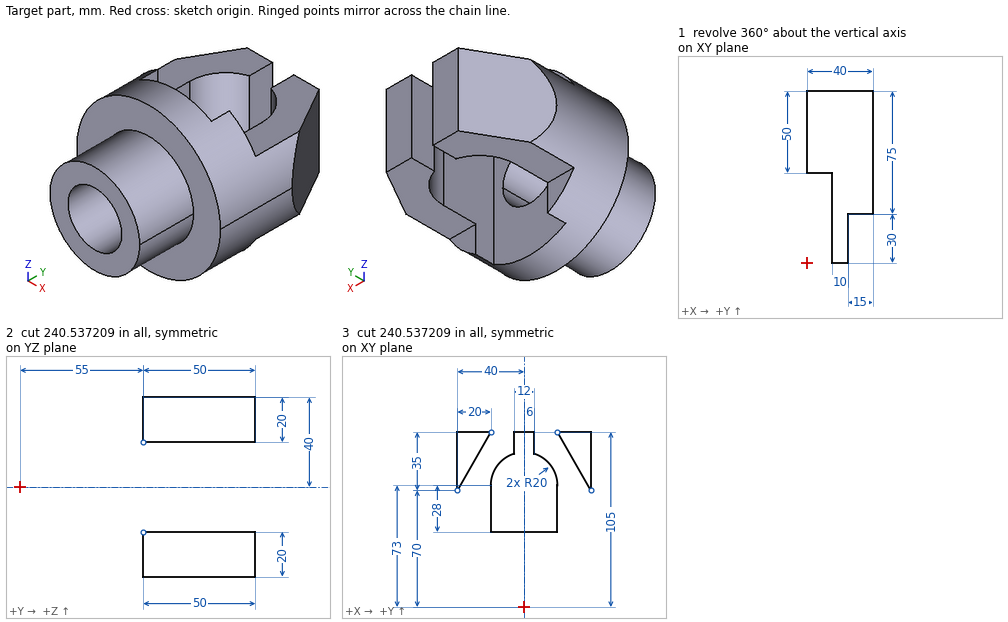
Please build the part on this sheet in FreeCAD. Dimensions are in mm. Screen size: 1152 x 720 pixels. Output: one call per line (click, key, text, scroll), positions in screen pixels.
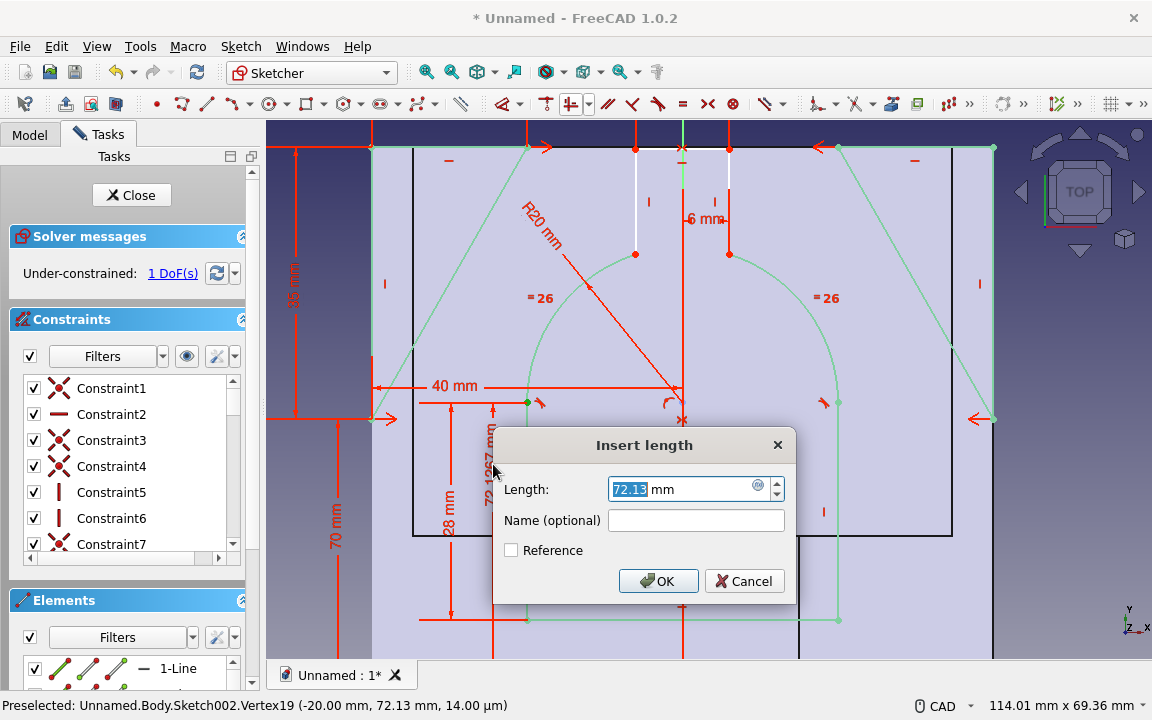
text(73)
key(Return)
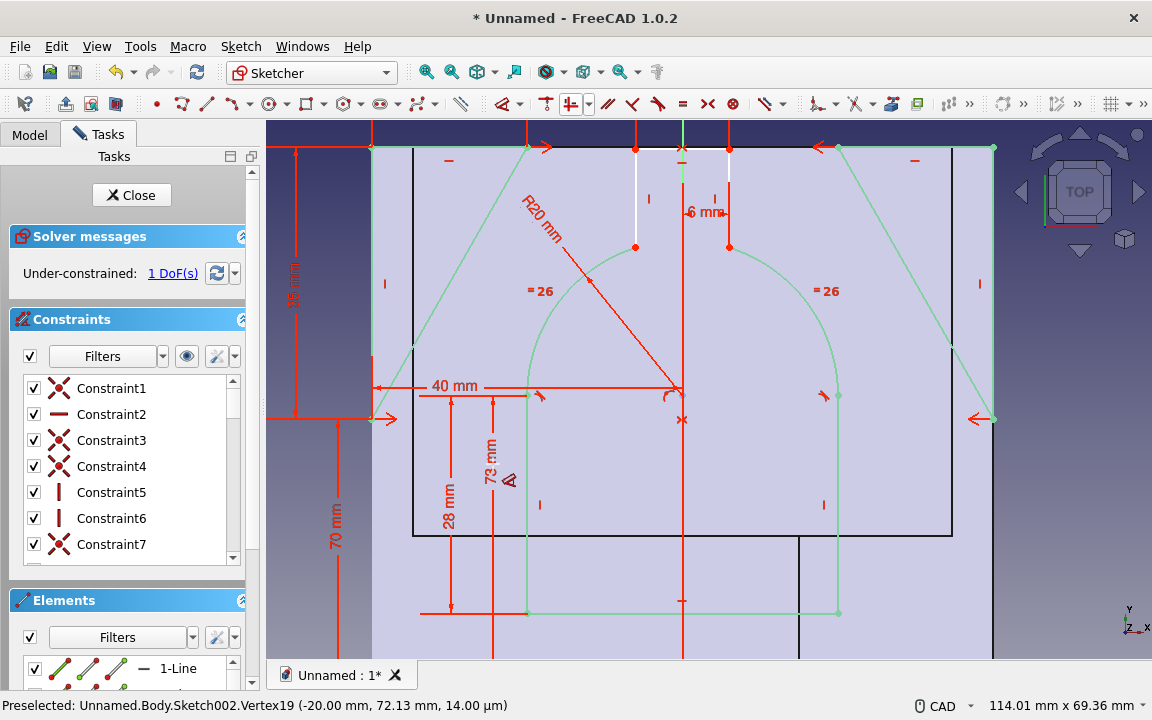
click(729, 149)
click(763, 390)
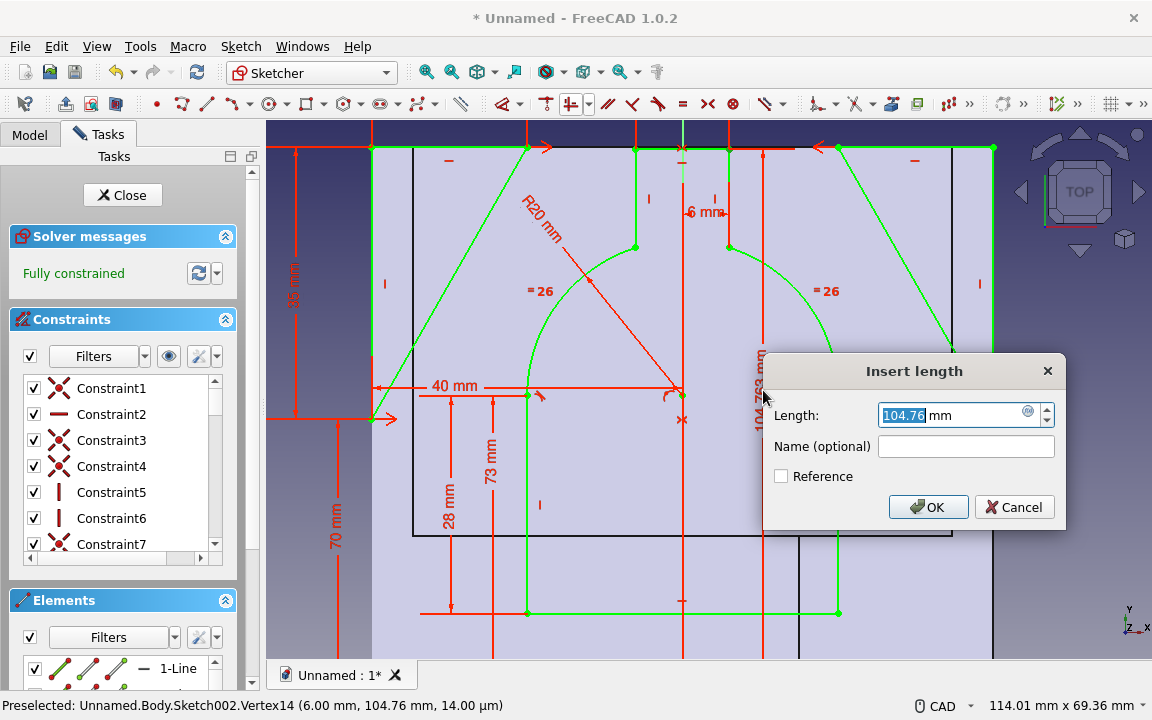
text(105)
key(Return)
key(Escape)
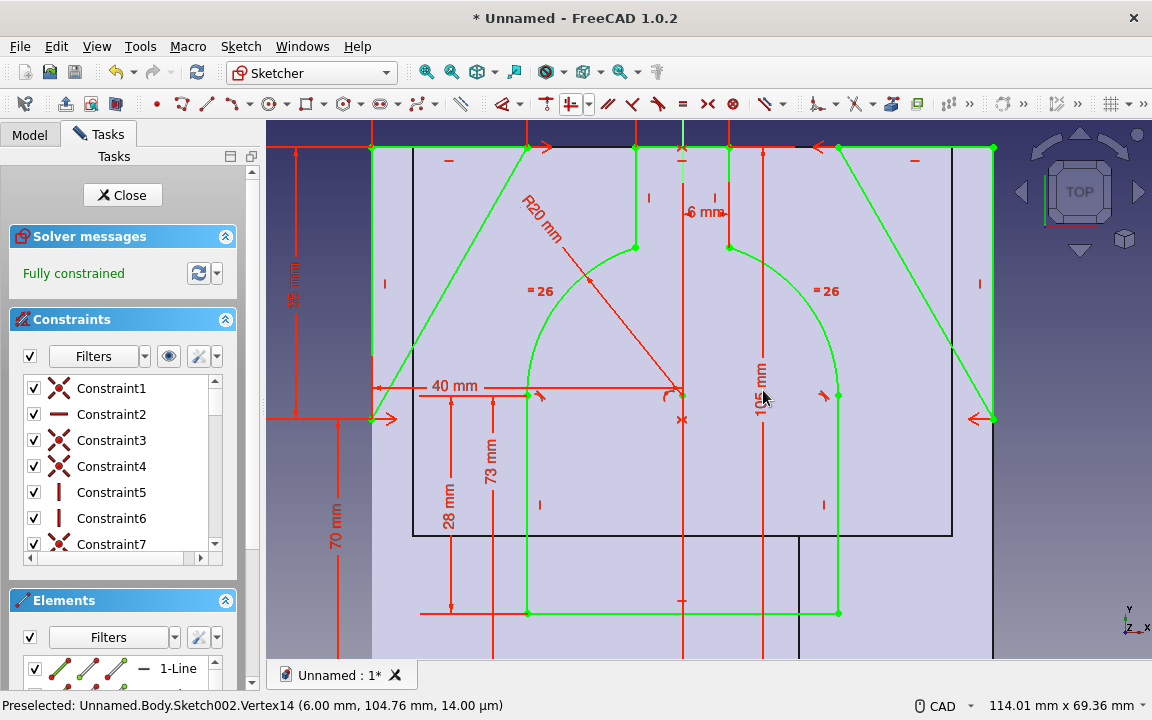
click(123, 195)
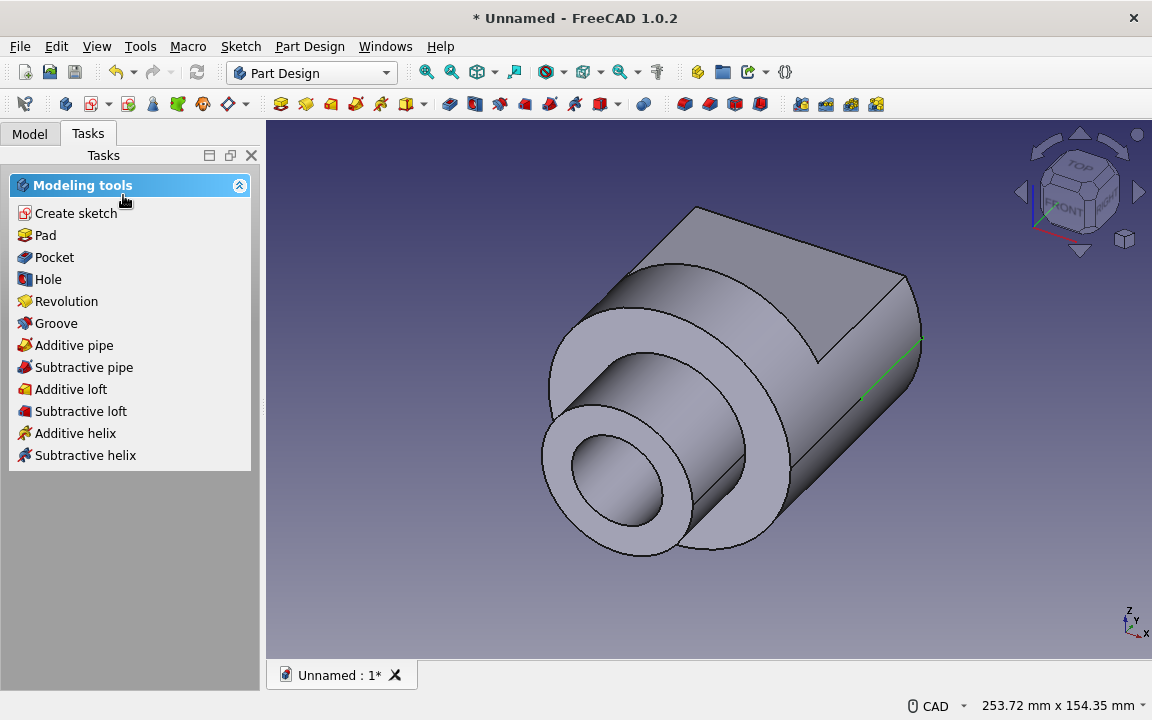
click(450, 104)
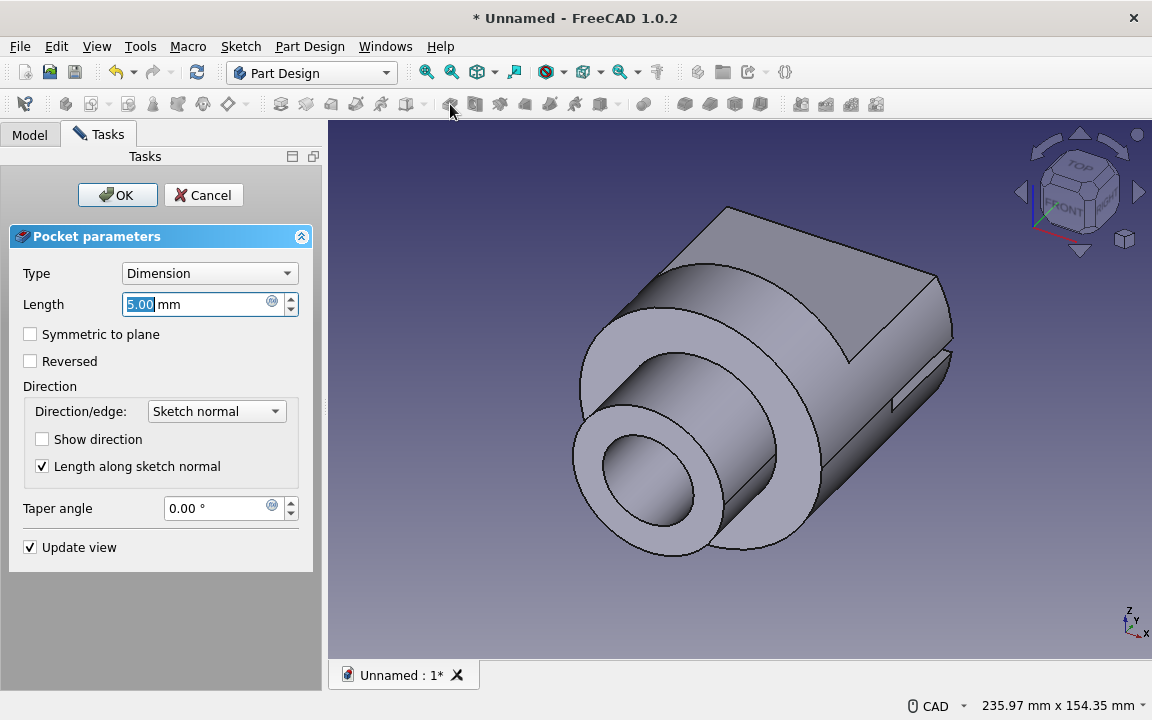
text(240.537209)
key(Tab)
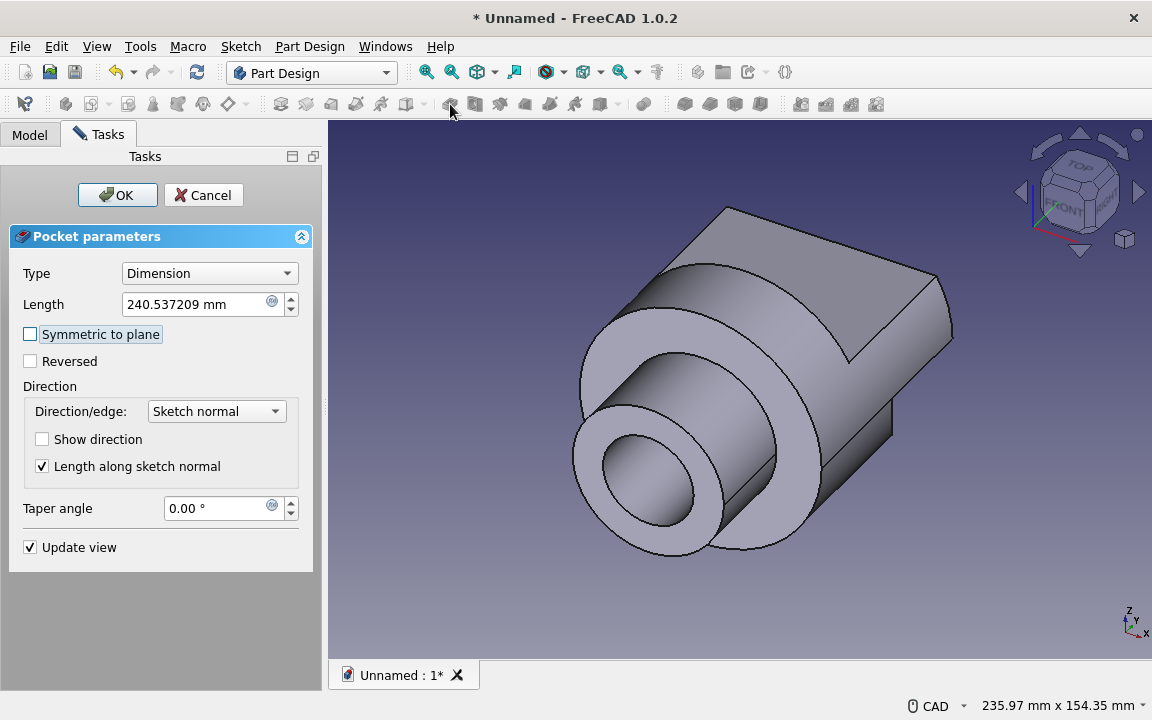
click(31, 334)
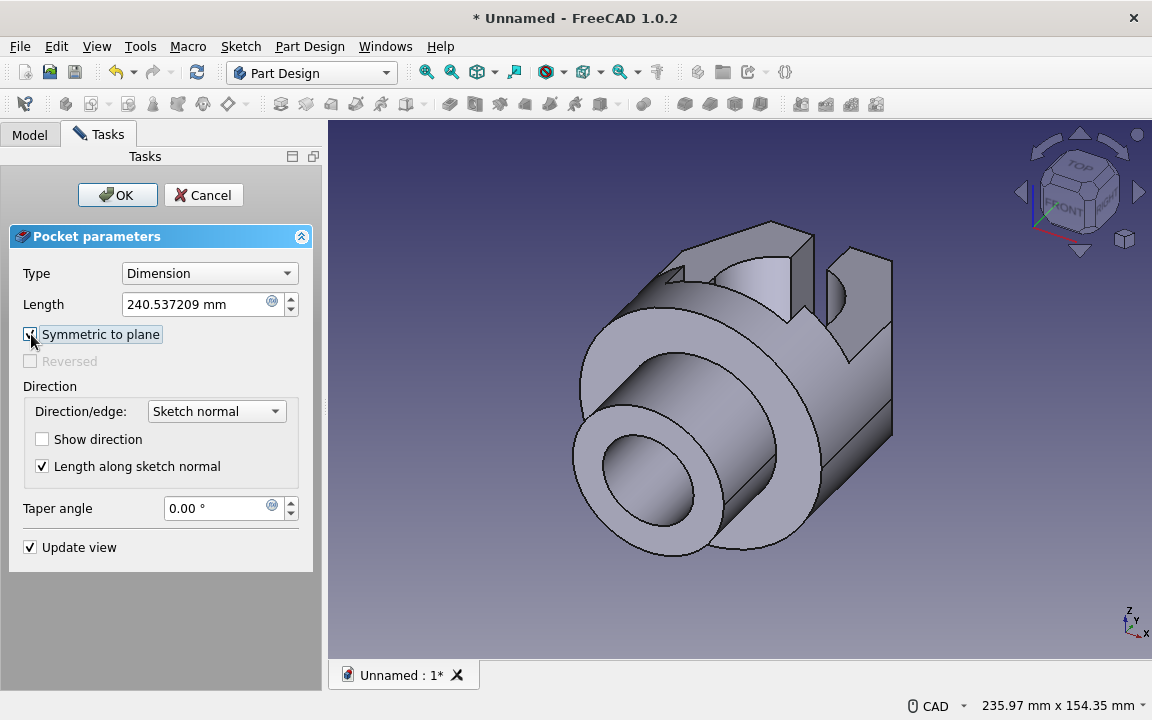
click(118, 195)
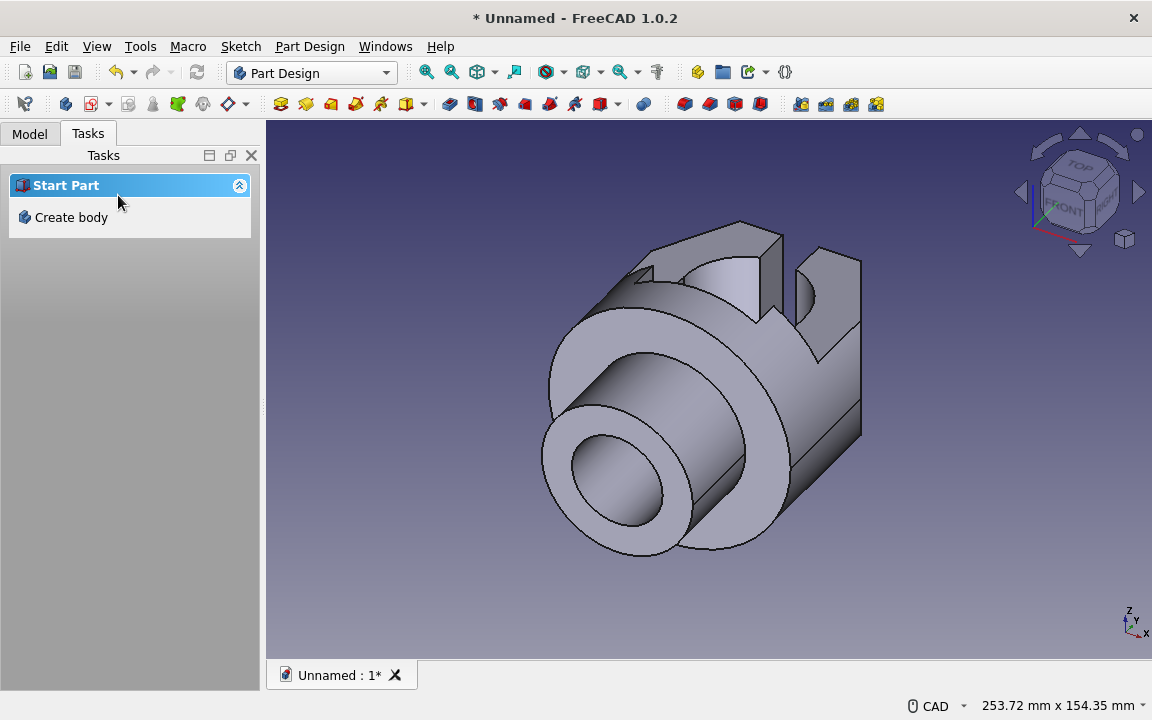
key(0)